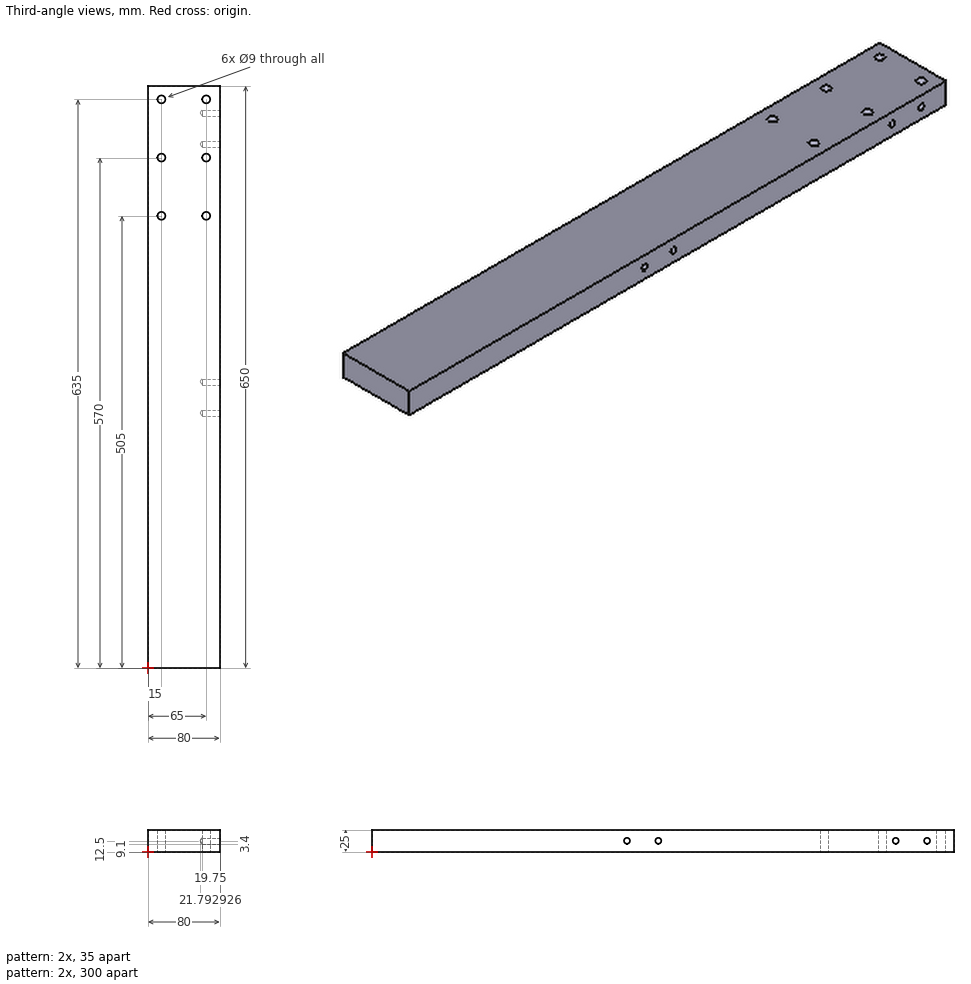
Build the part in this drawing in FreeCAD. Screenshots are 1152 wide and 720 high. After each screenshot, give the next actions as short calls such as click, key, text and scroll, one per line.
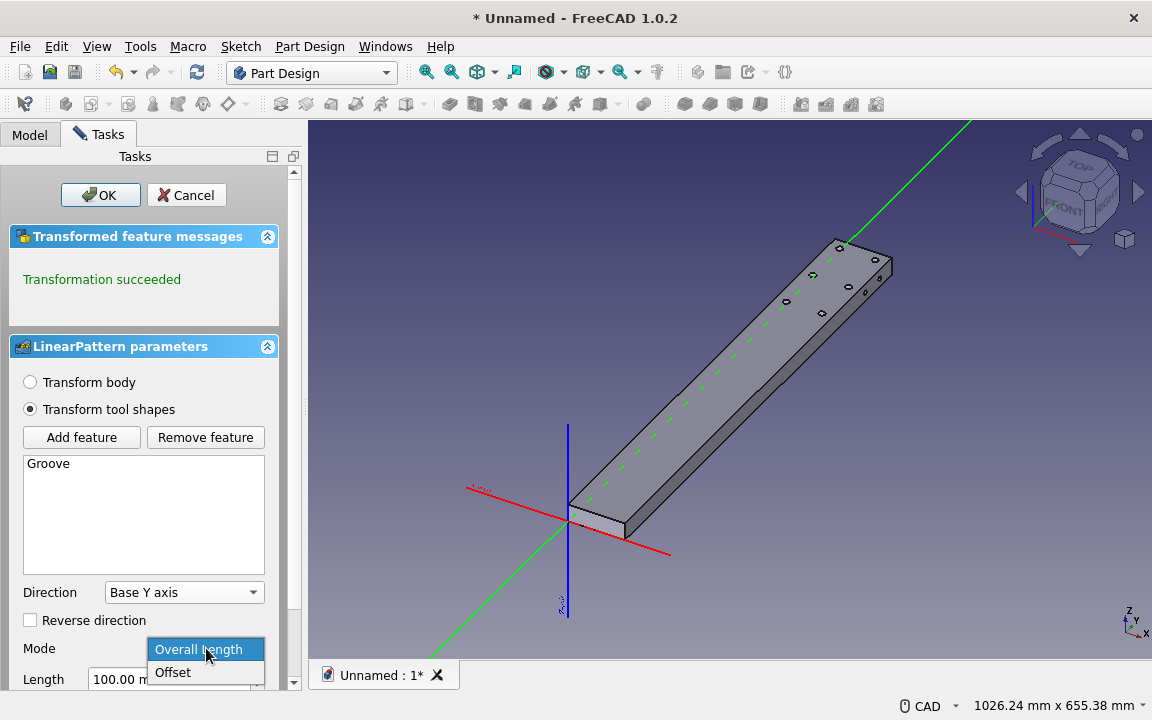
click(204, 672)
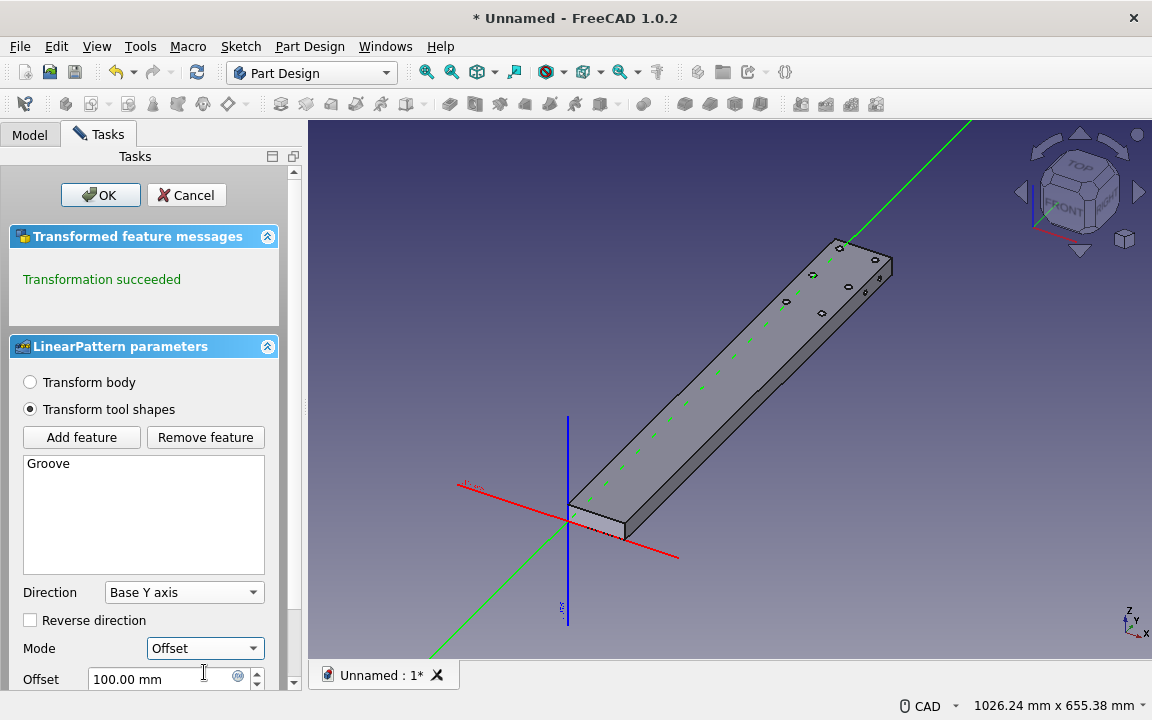
scroll(294, 428, down, 2)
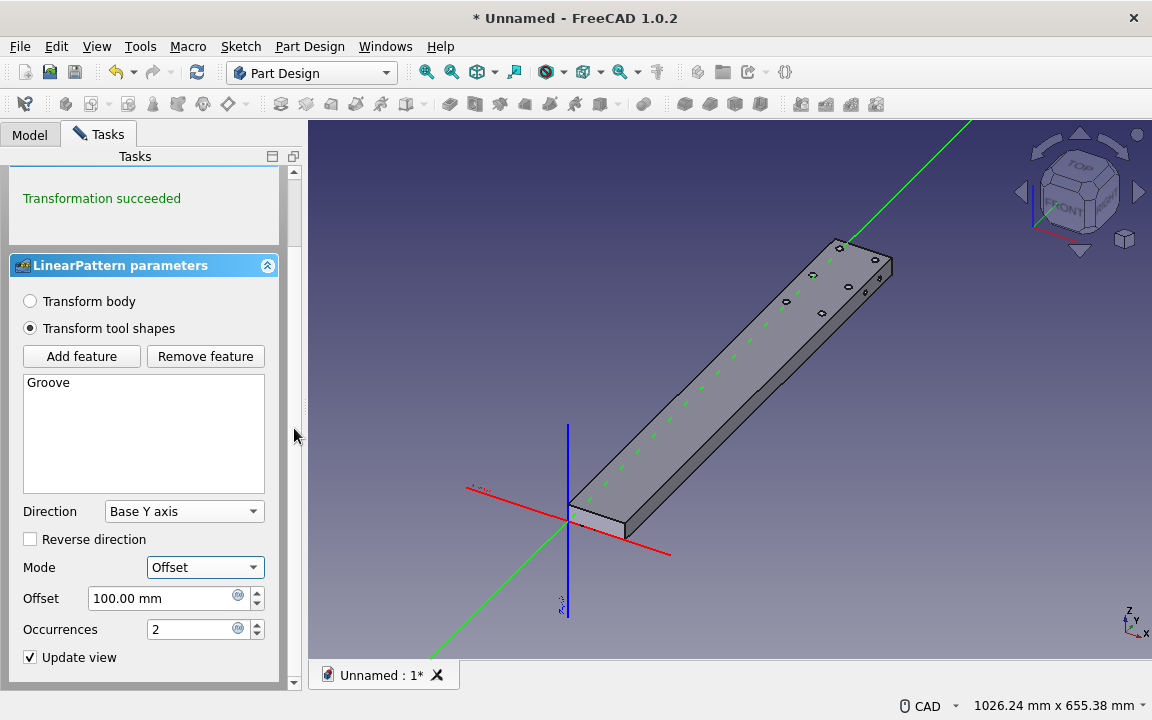
triple_click(170, 598)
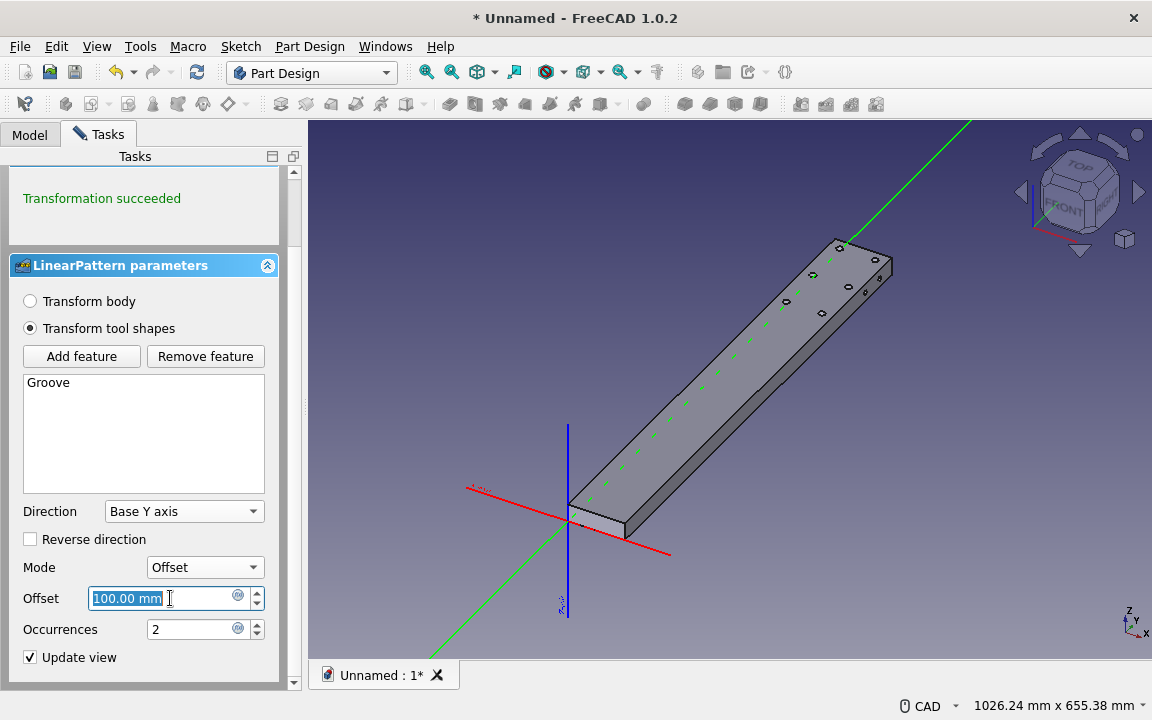
text(300)
key(Tab)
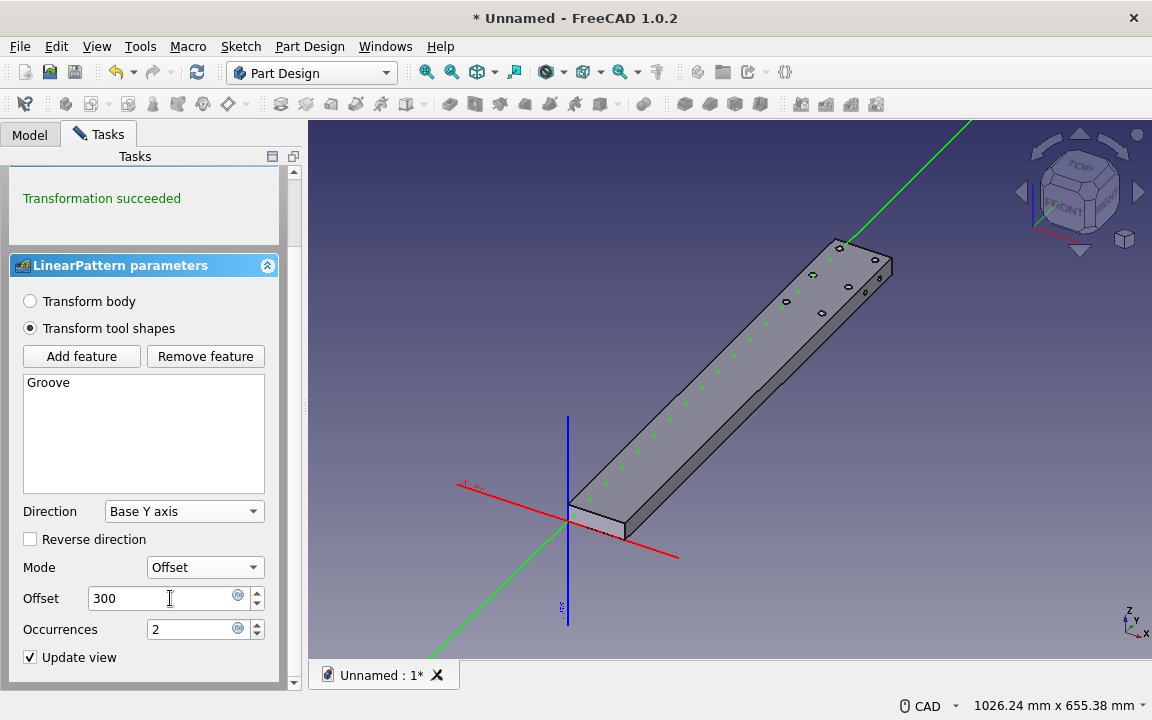
triple_click(199, 630)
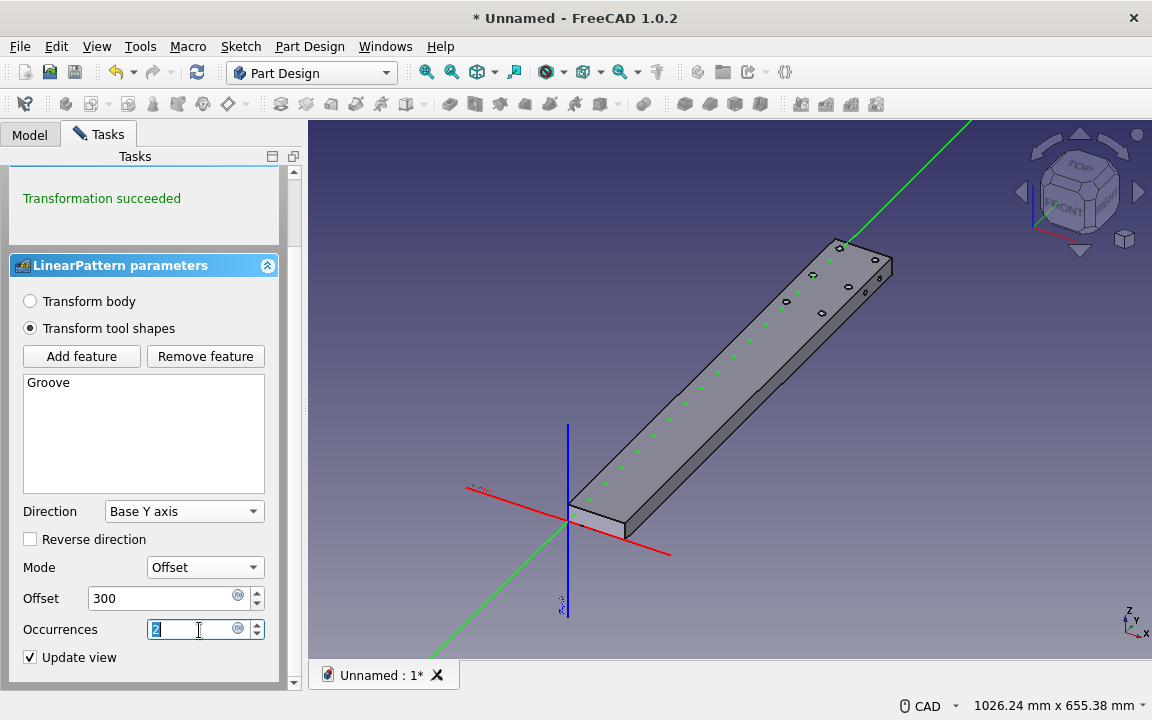
text(2)
key(Tab)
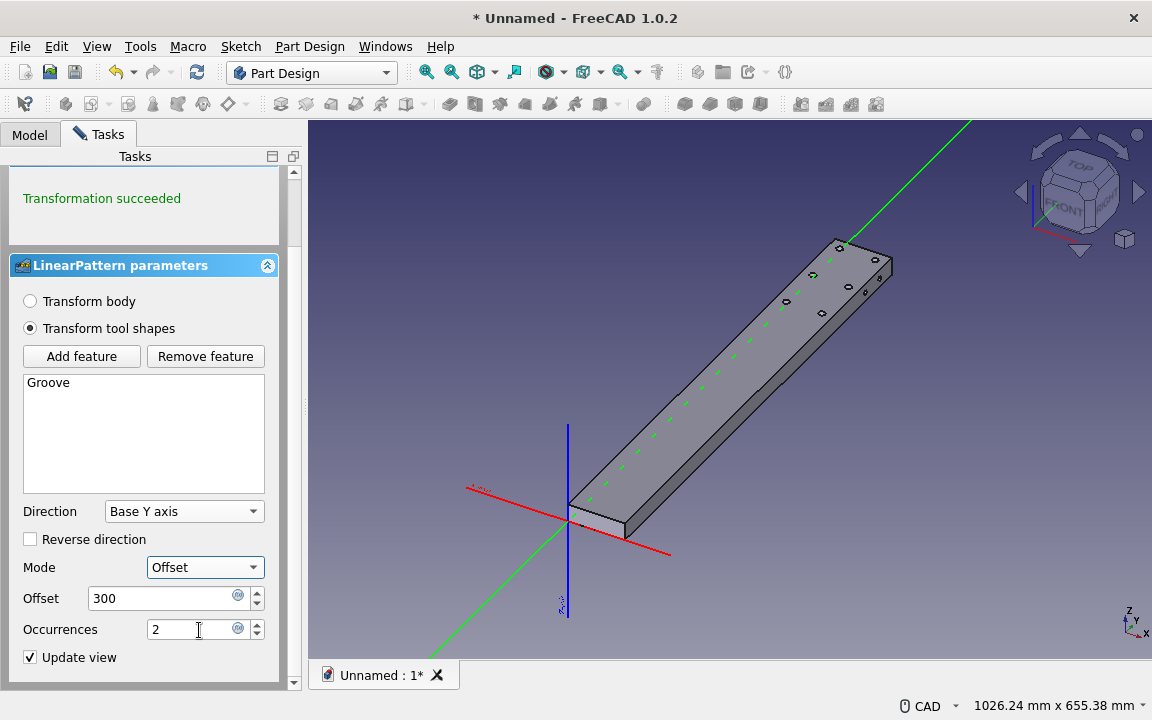
click(31, 539)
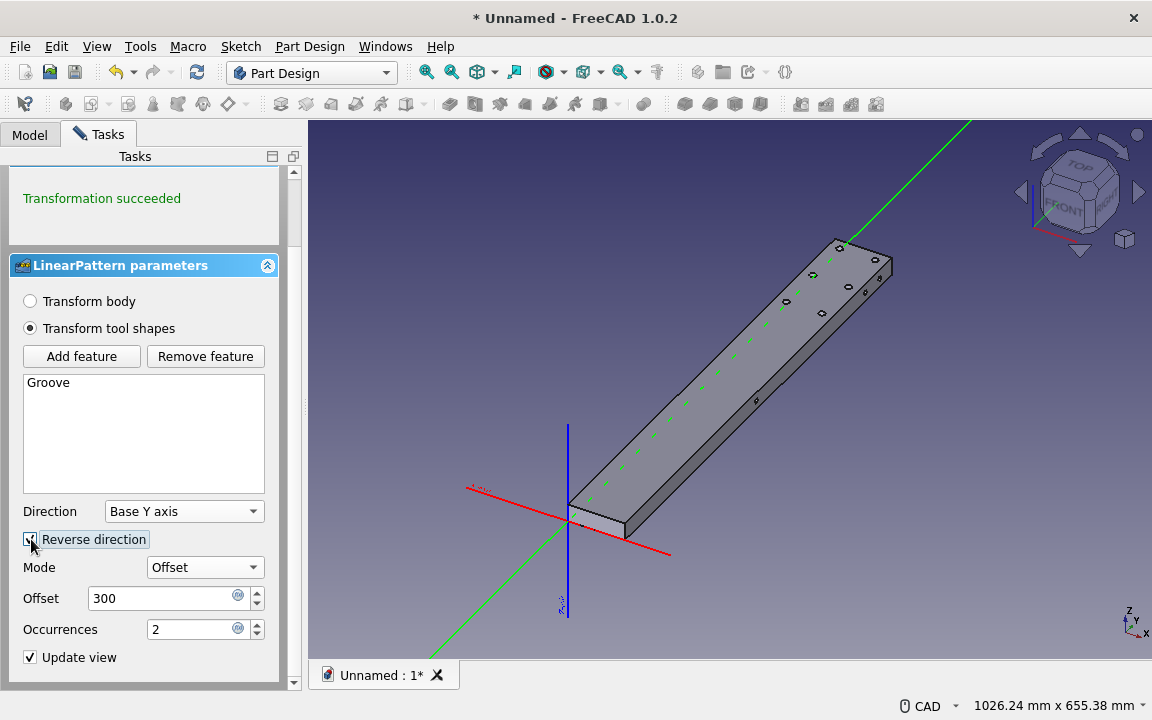
scroll(294, 428, up, 3)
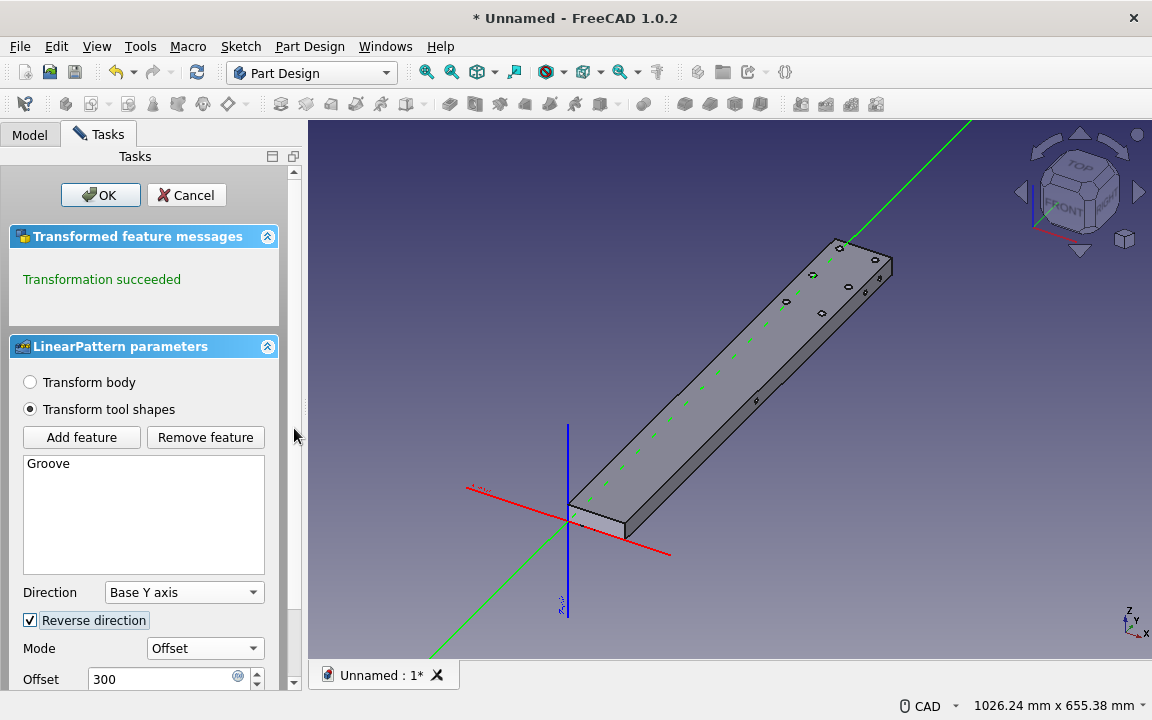
click(101, 195)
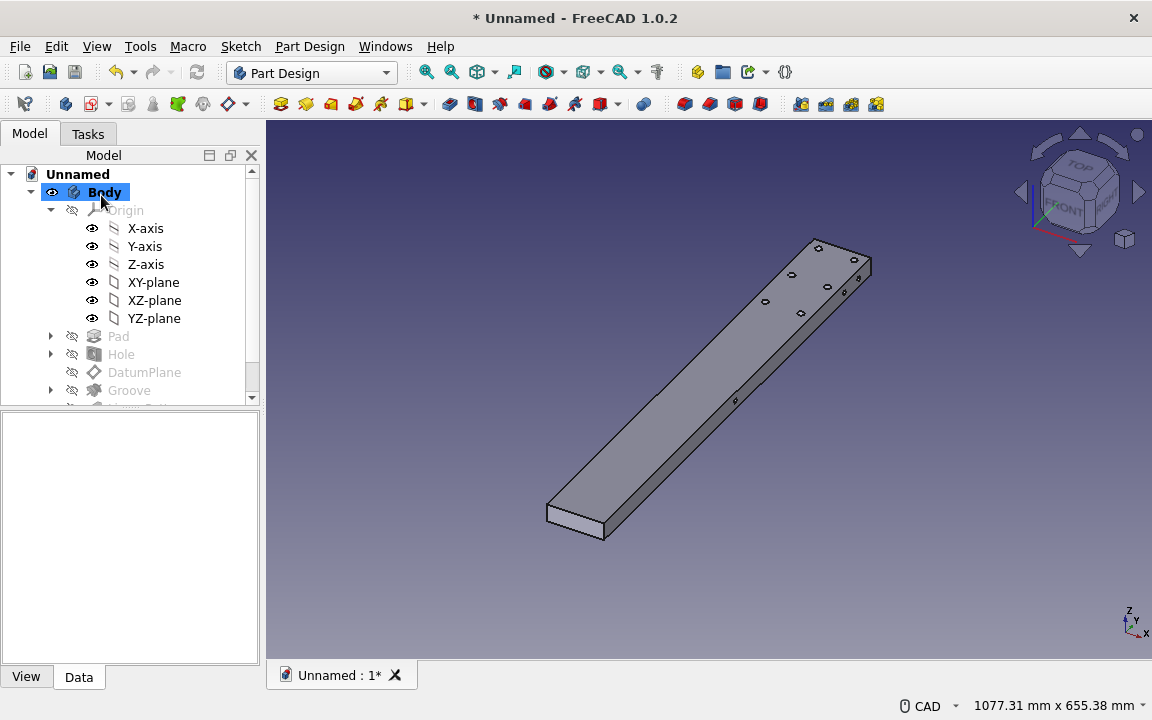
click(137, 300)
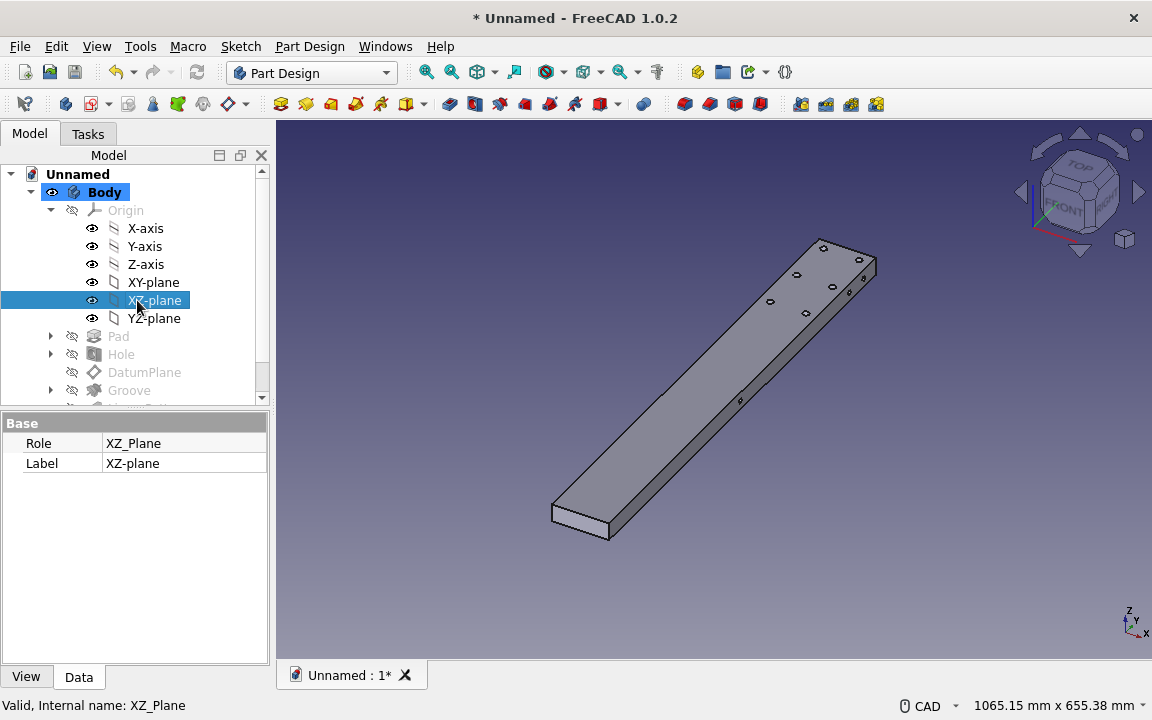
click(228, 104)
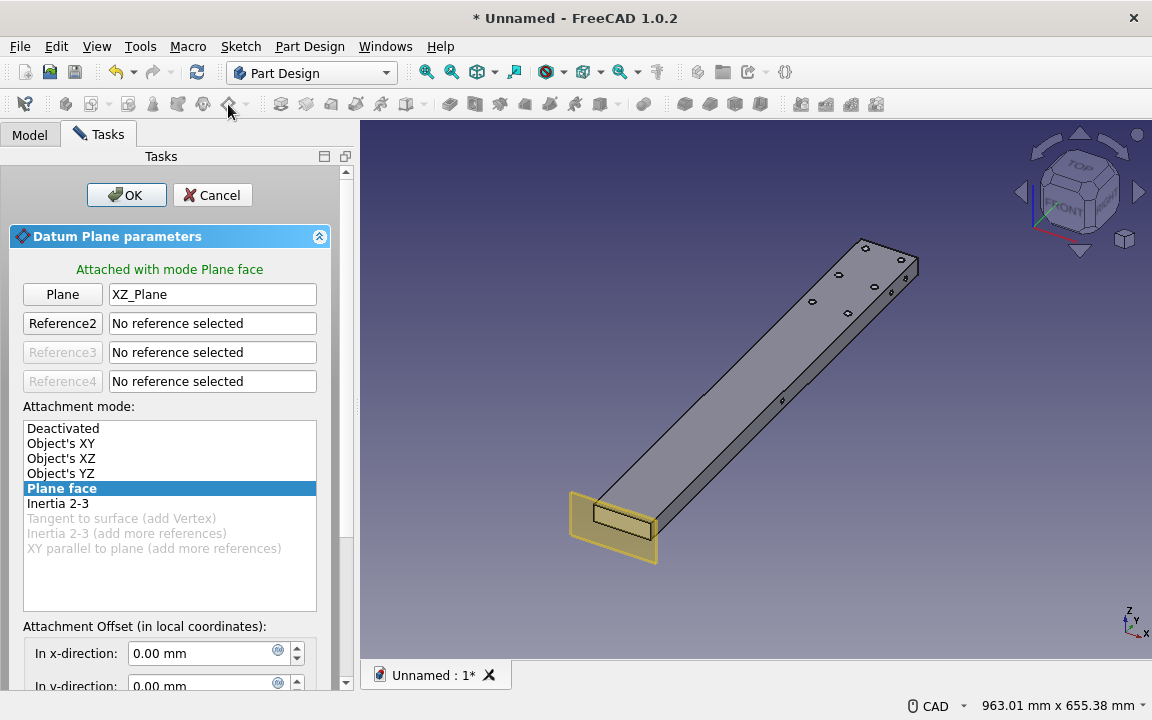
scroll(346, 428, down, 2)